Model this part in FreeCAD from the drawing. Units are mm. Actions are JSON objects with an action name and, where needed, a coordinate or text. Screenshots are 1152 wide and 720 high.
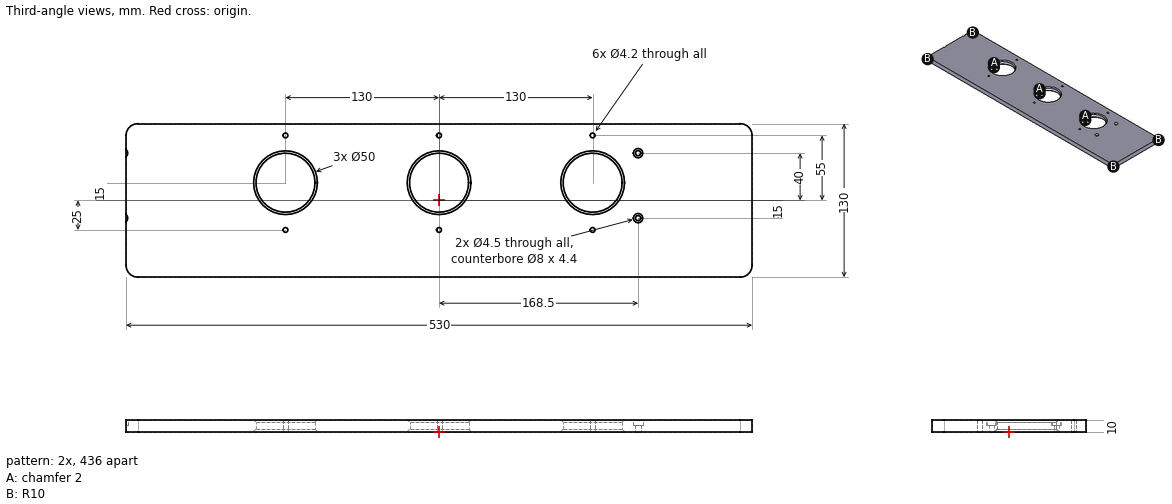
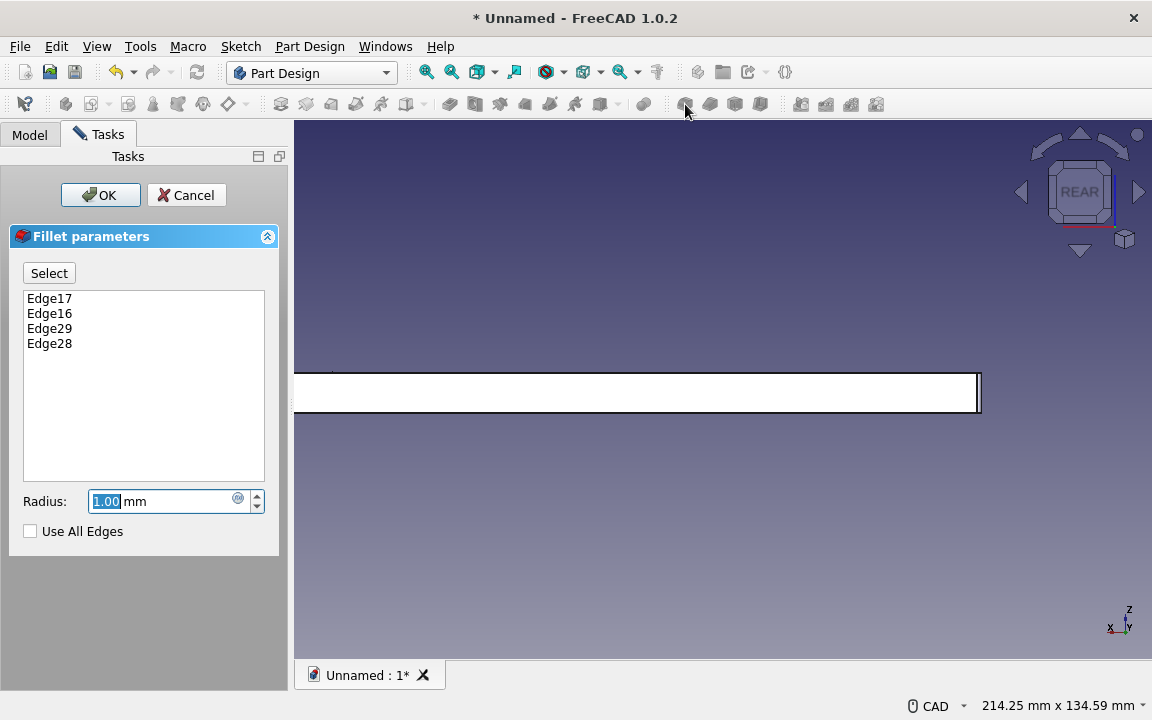
{"action": "type", "text": "10"}
{"action": "key", "text": "Tab"}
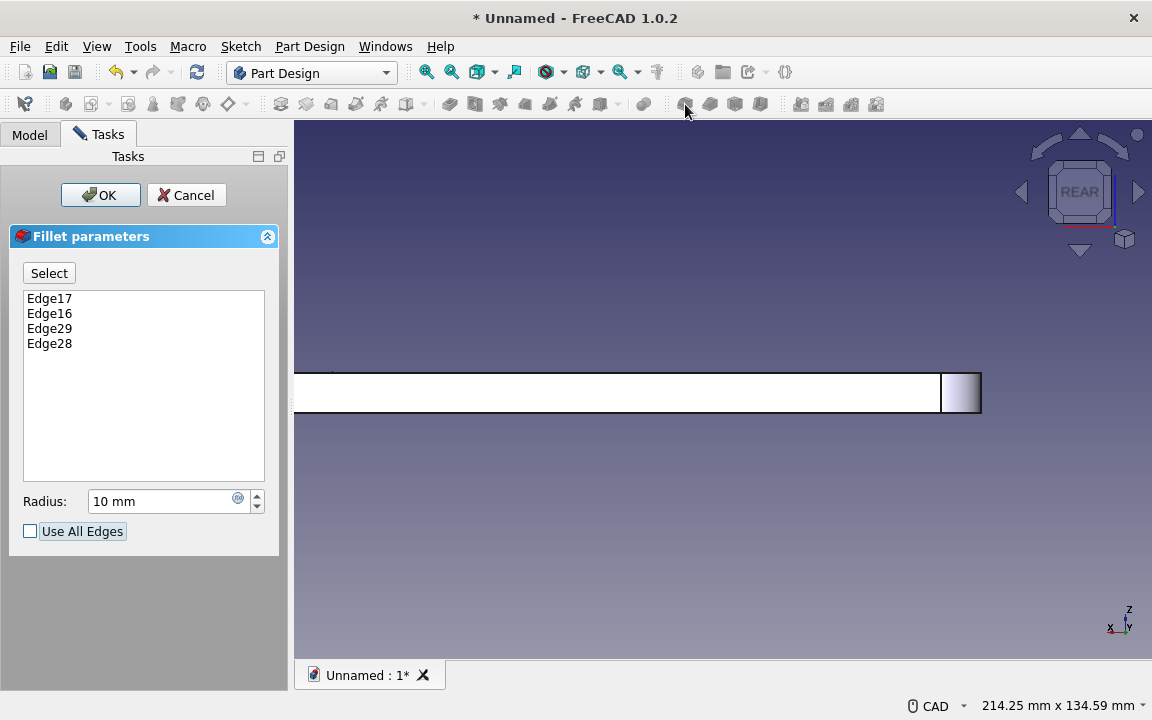
{"action": "left_click", "coordinate": [101, 195]}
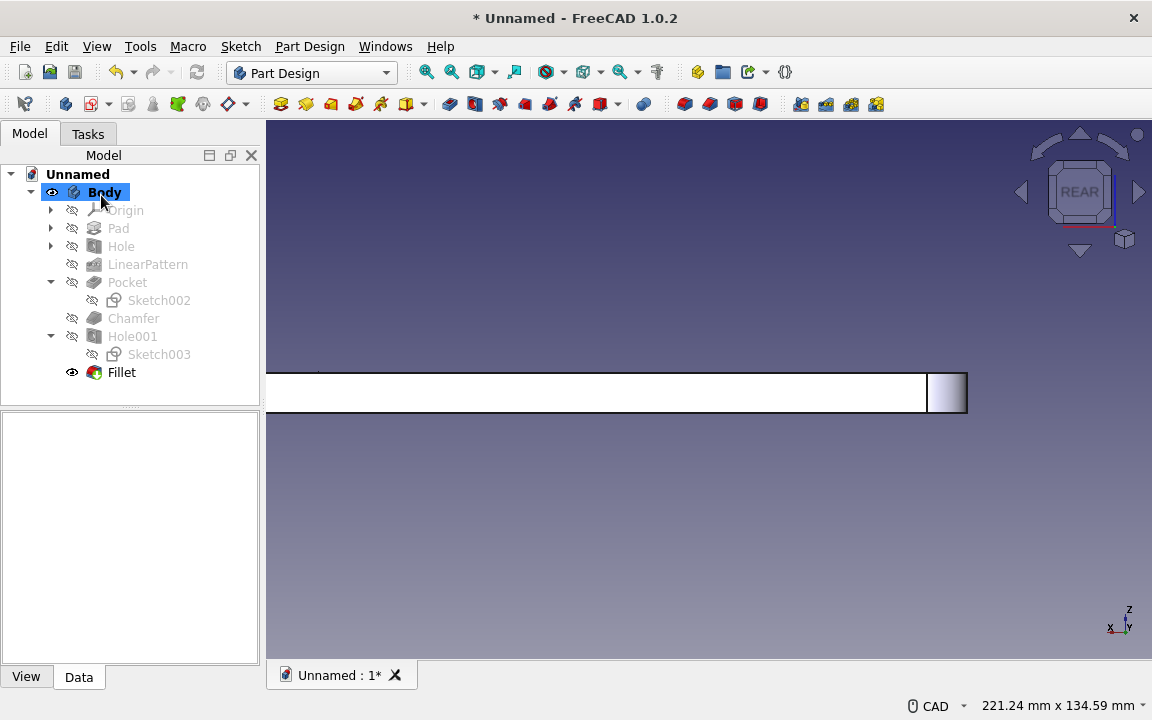
{"action": "key", "text": "0"}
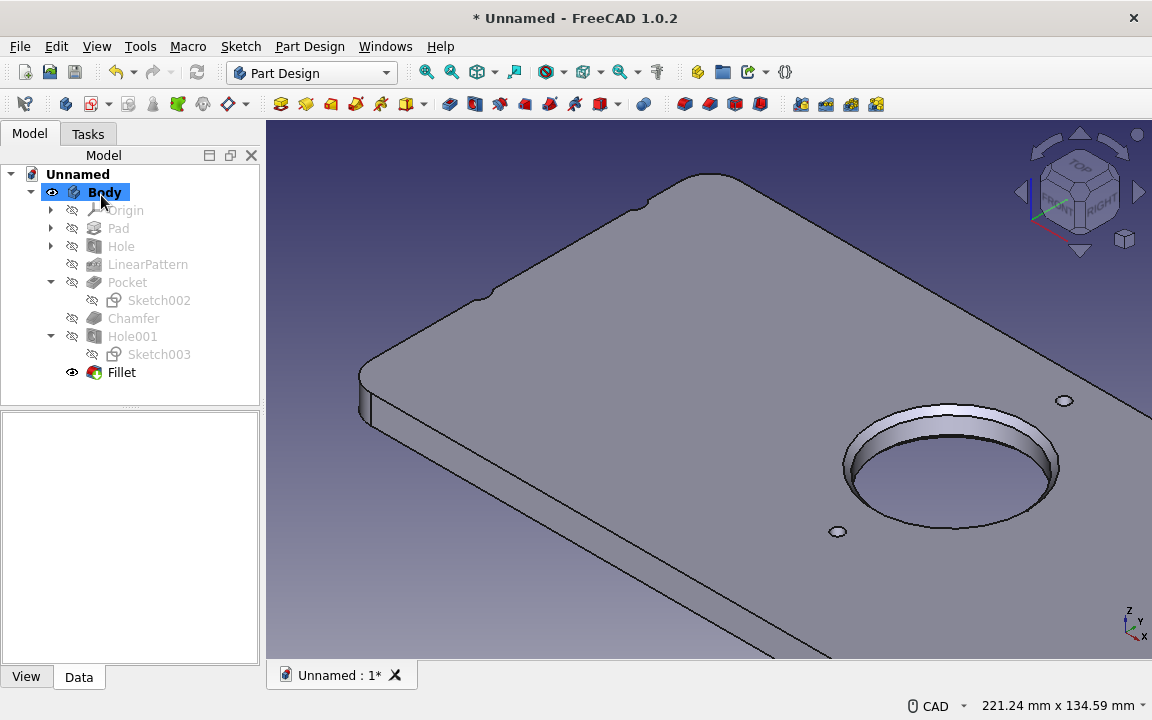
{"action": "left_click", "coordinate": [427, 72]}